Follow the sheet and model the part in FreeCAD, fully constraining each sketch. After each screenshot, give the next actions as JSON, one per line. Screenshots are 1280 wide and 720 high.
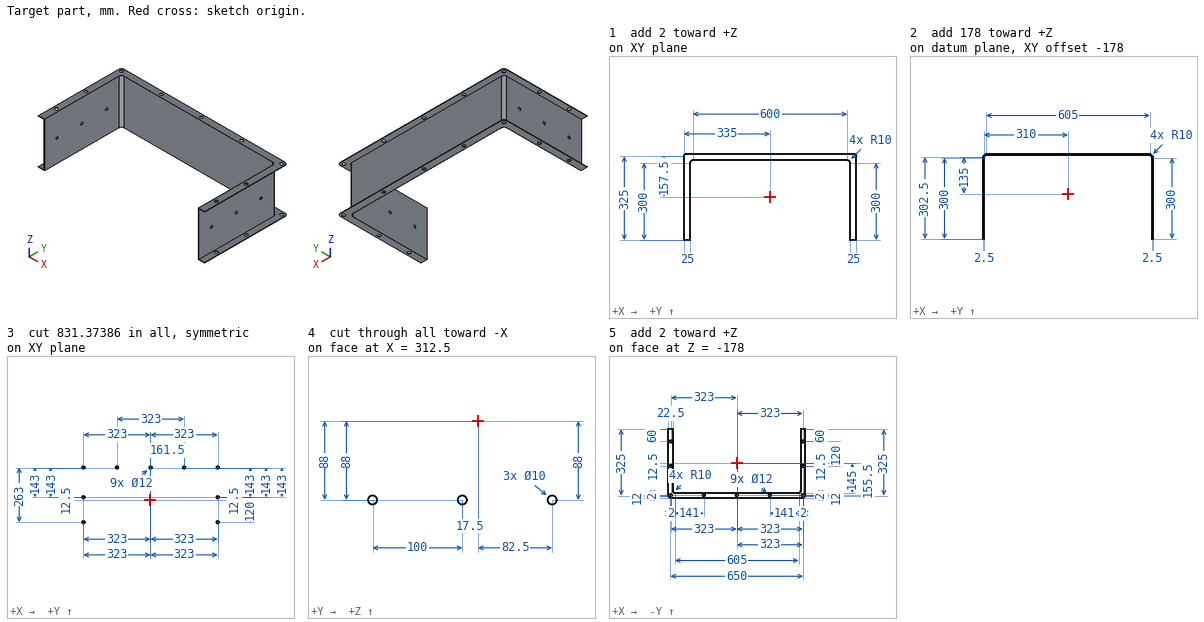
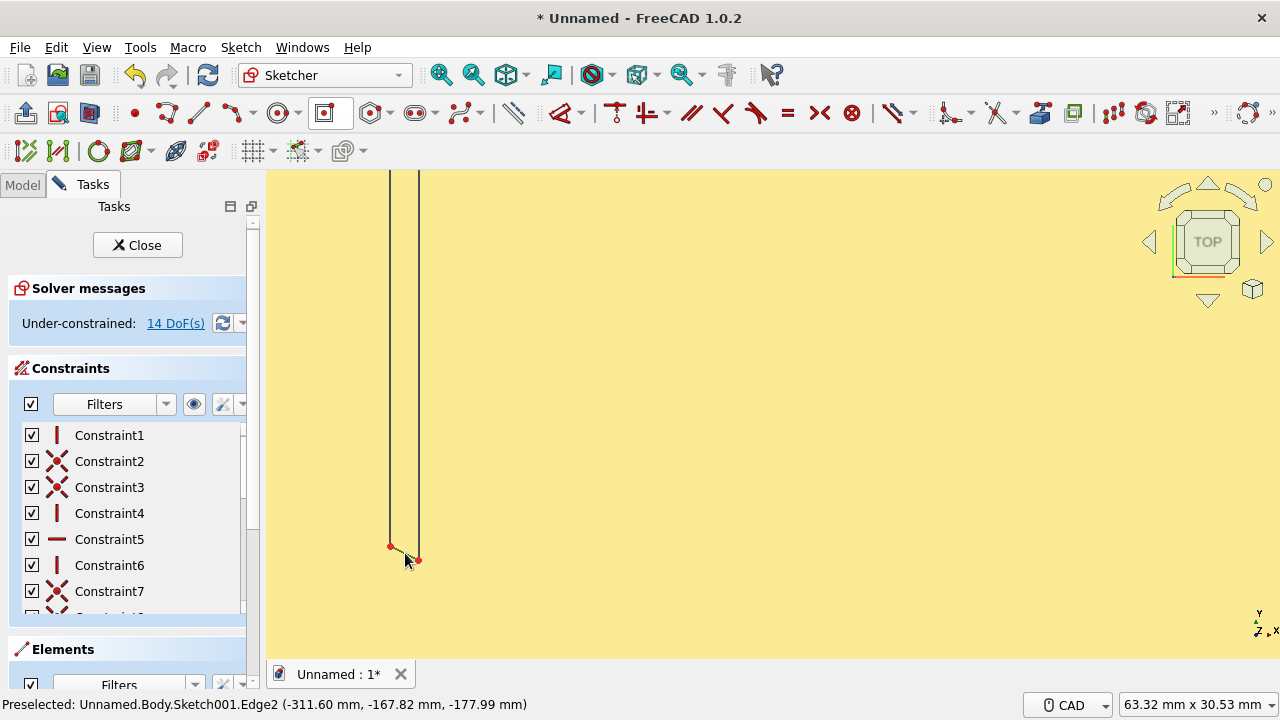
{"action": "left_click", "coordinate": [670, 114]}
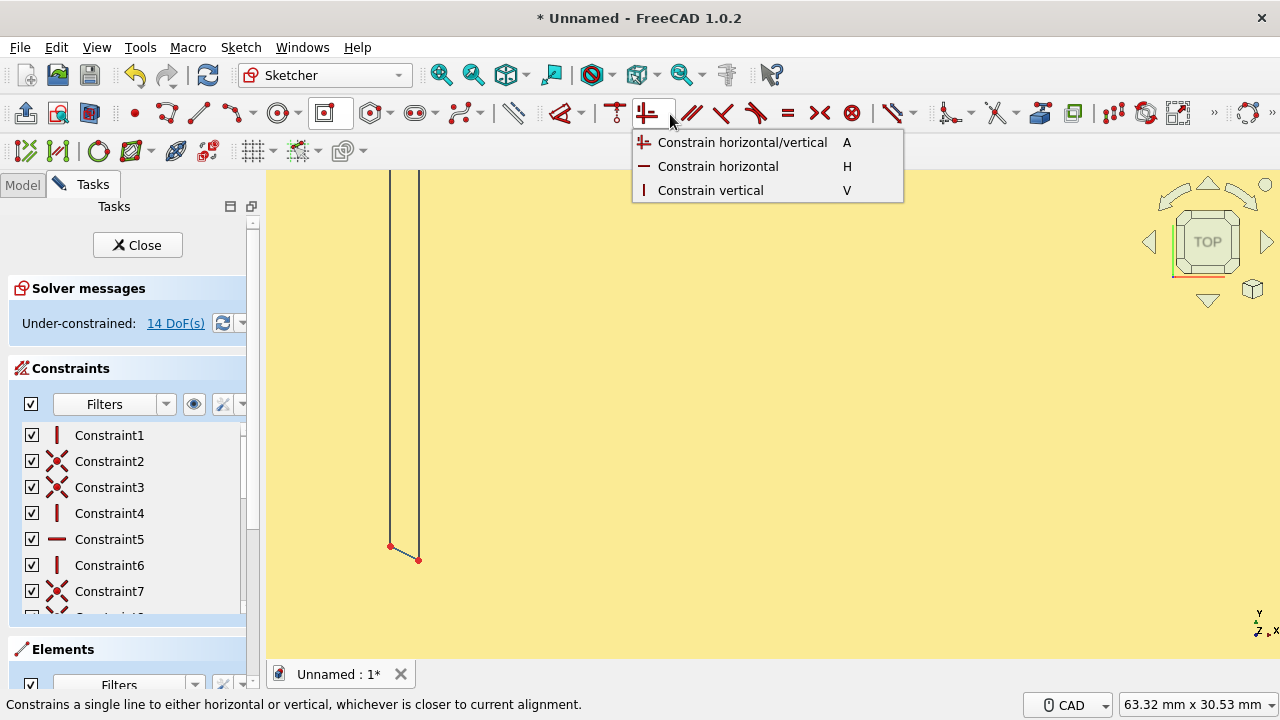
{"action": "left_click", "coordinate": [768, 166]}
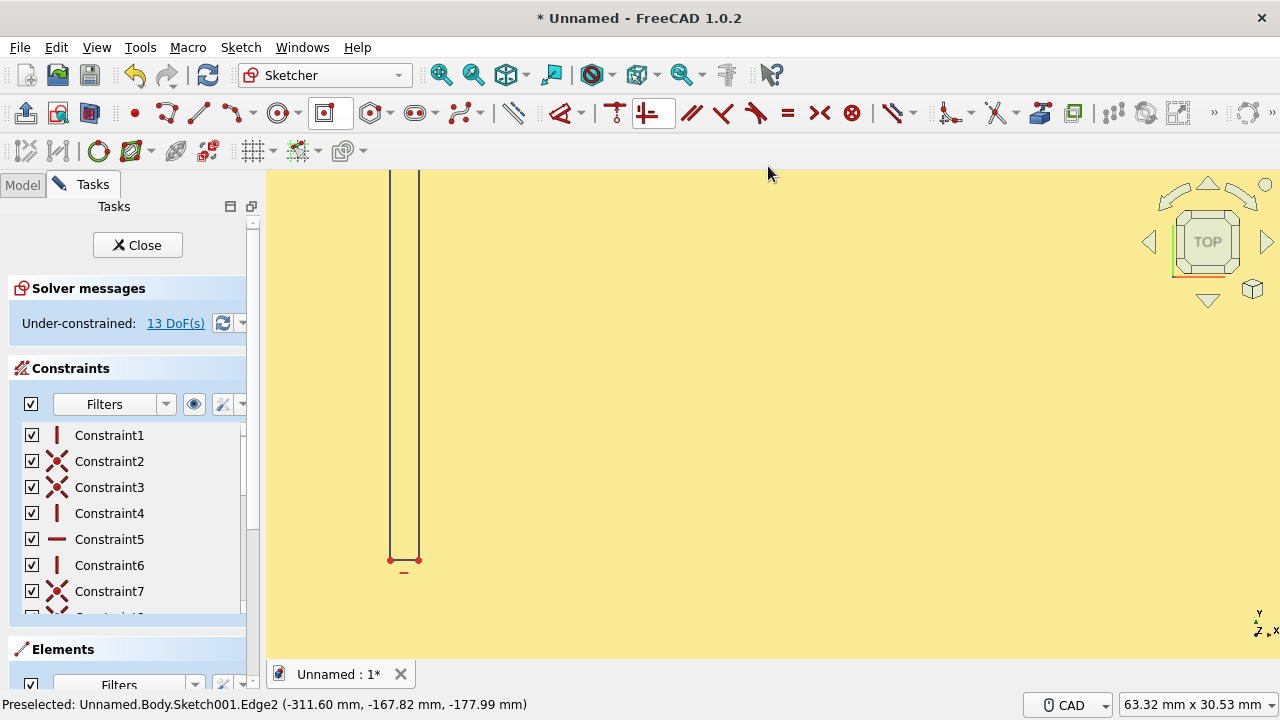
{"action": "scroll", "coordinate": [401, 568], "scroll_direction": "down", "scroll_amount": 14}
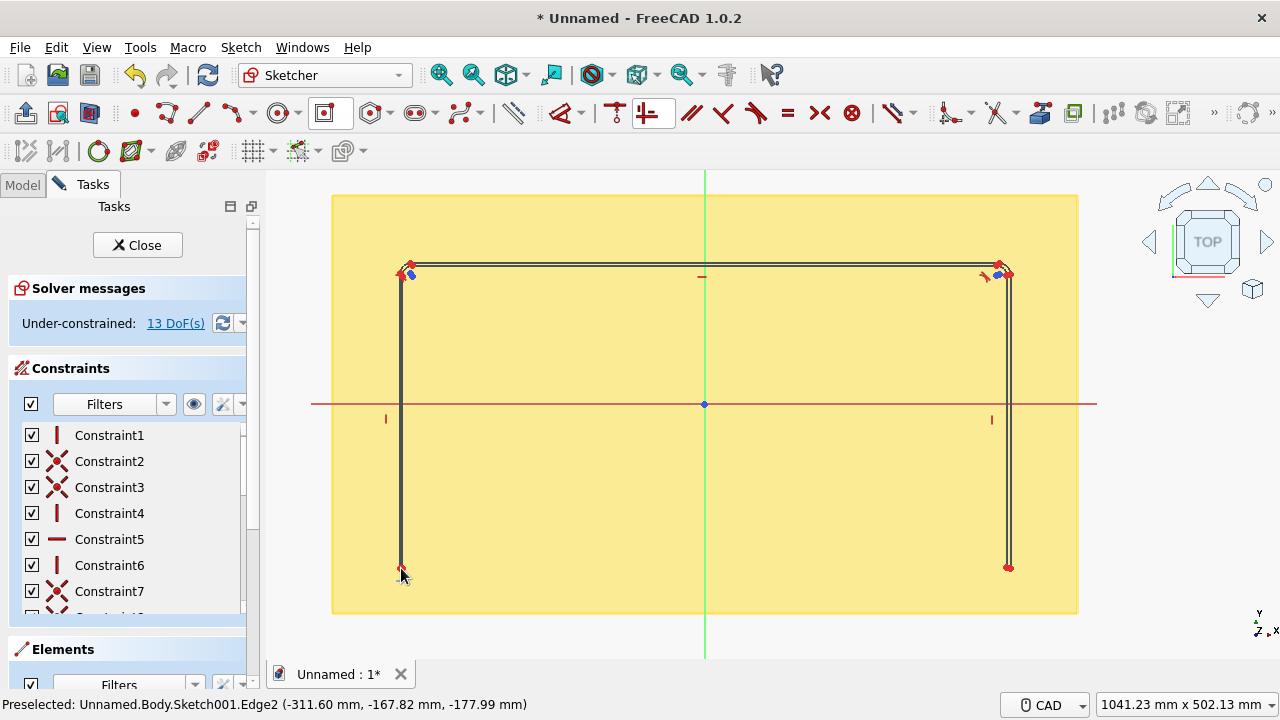
{"action": "scroll", "coordinate": [1009, 568], "scroll_direction": "up", "scroll_amount": 13}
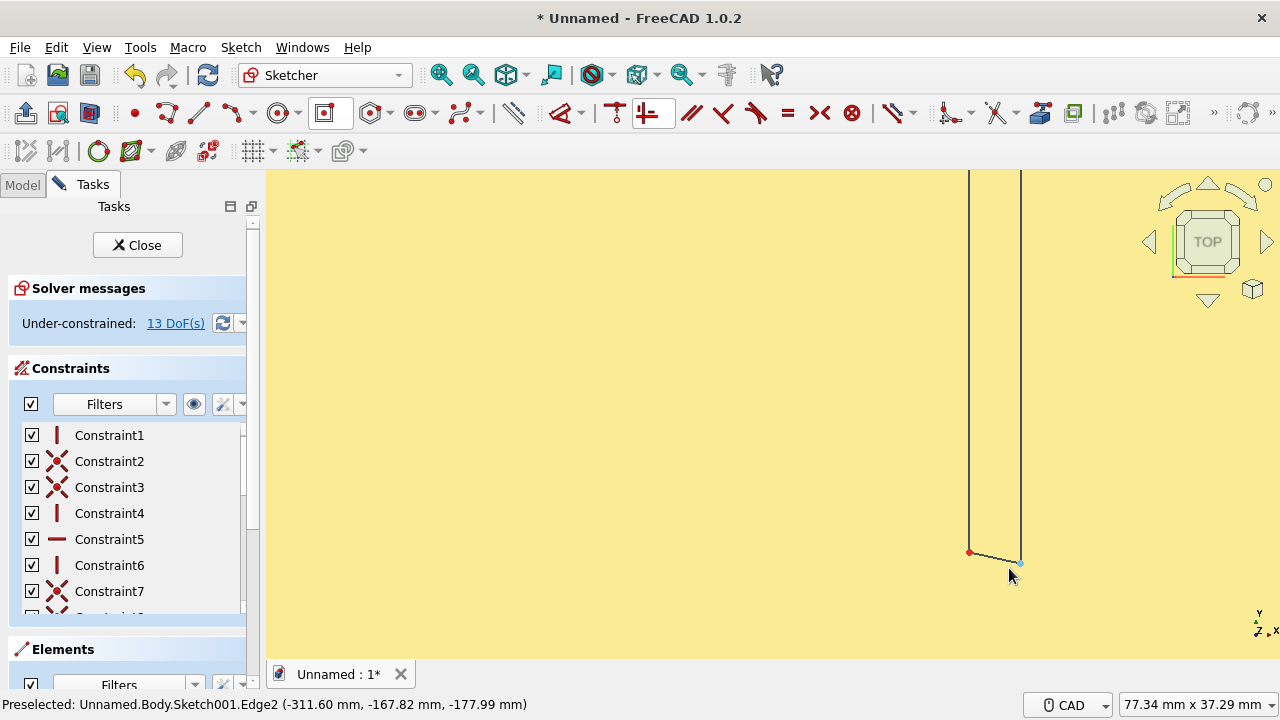
{"action": "left_click", "coordinate": [1005, 560]}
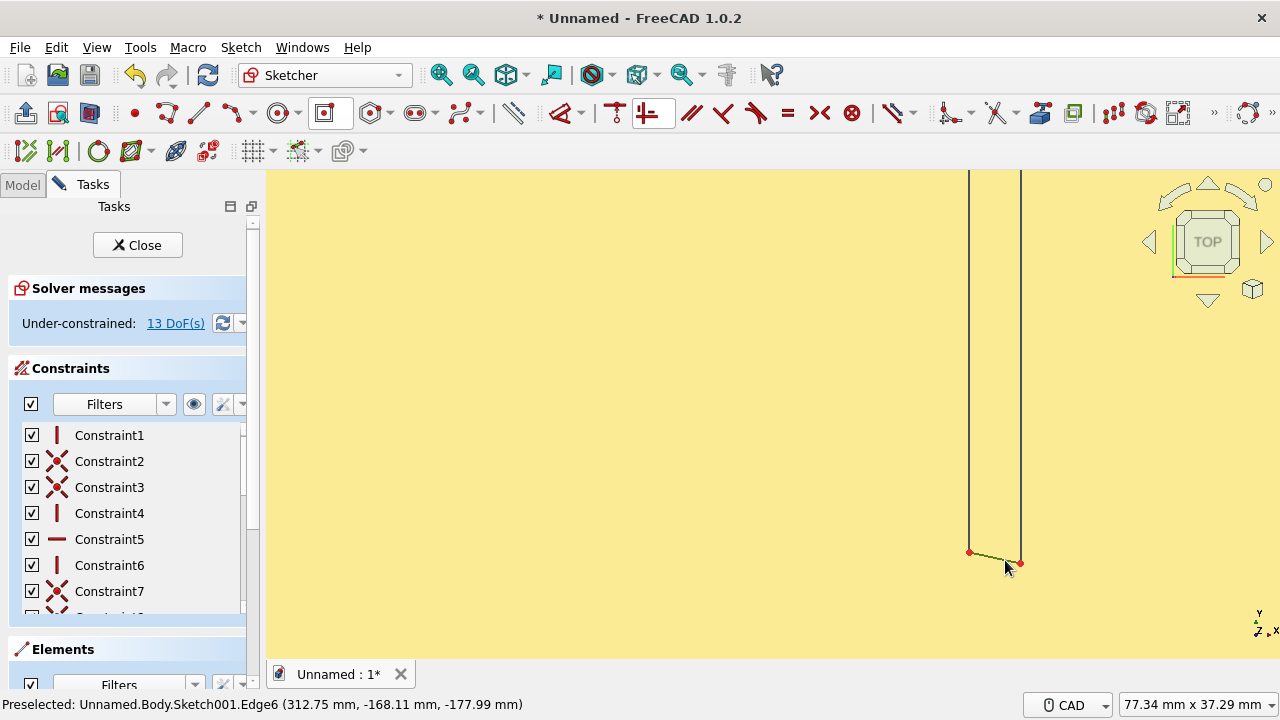
{"action": "left_click", "coordinate": [670, 114]}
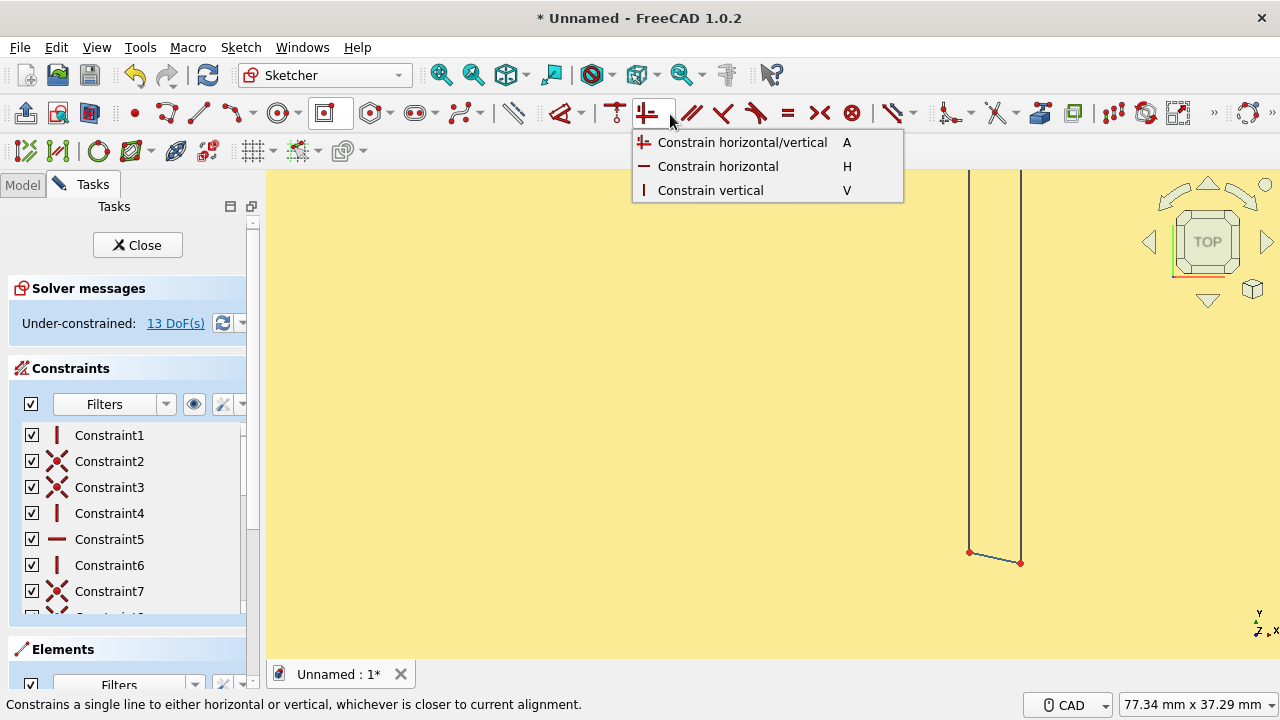
{"action": "left_click", "coordinate": [768, 166]}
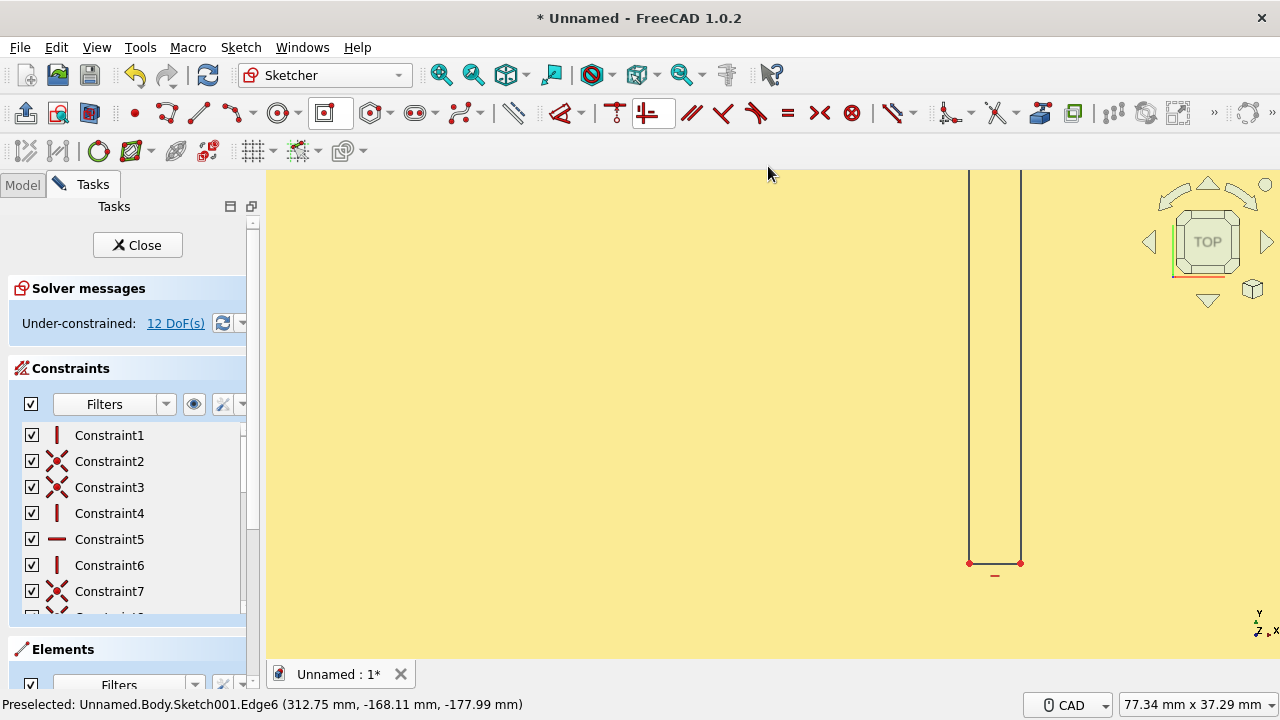
{"action": "scroll", "coordinate": [1009, 568], "scroll_direction": "down", "scroll_amount": 13}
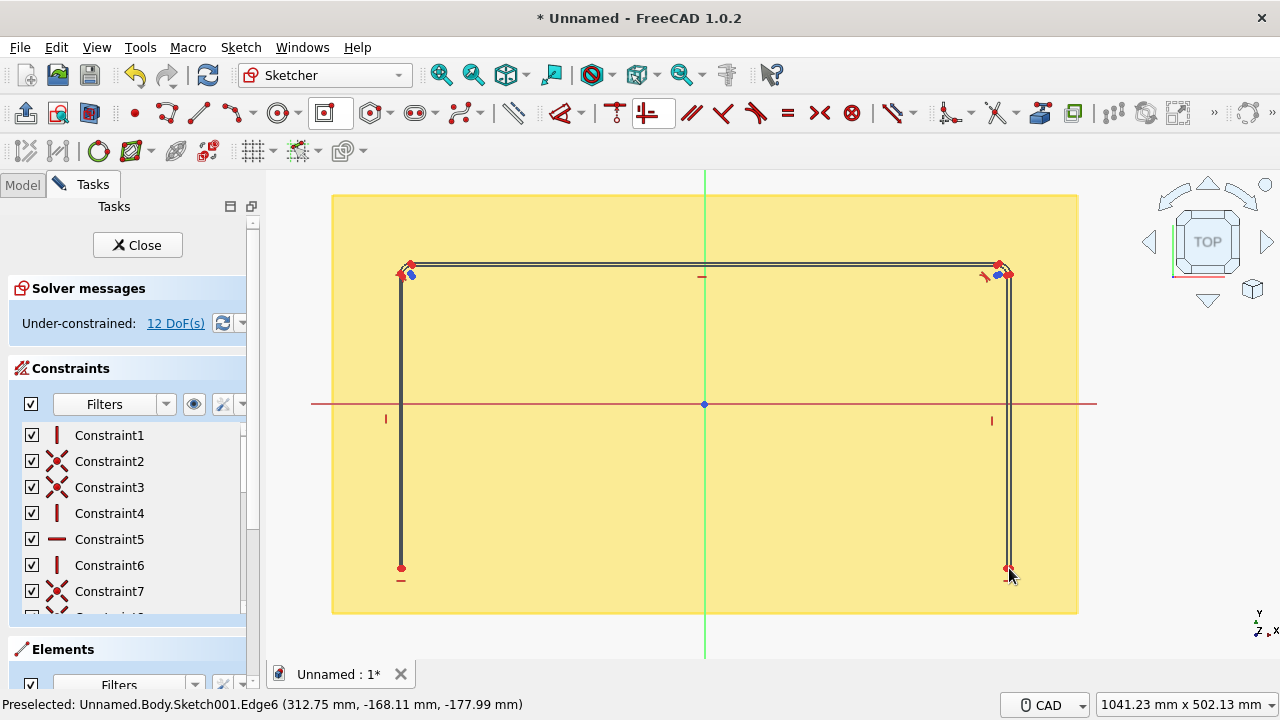
{"action": "scroll", "coordinate": [406, 264], "scroll_direction": "up", "scroll_amount": 8}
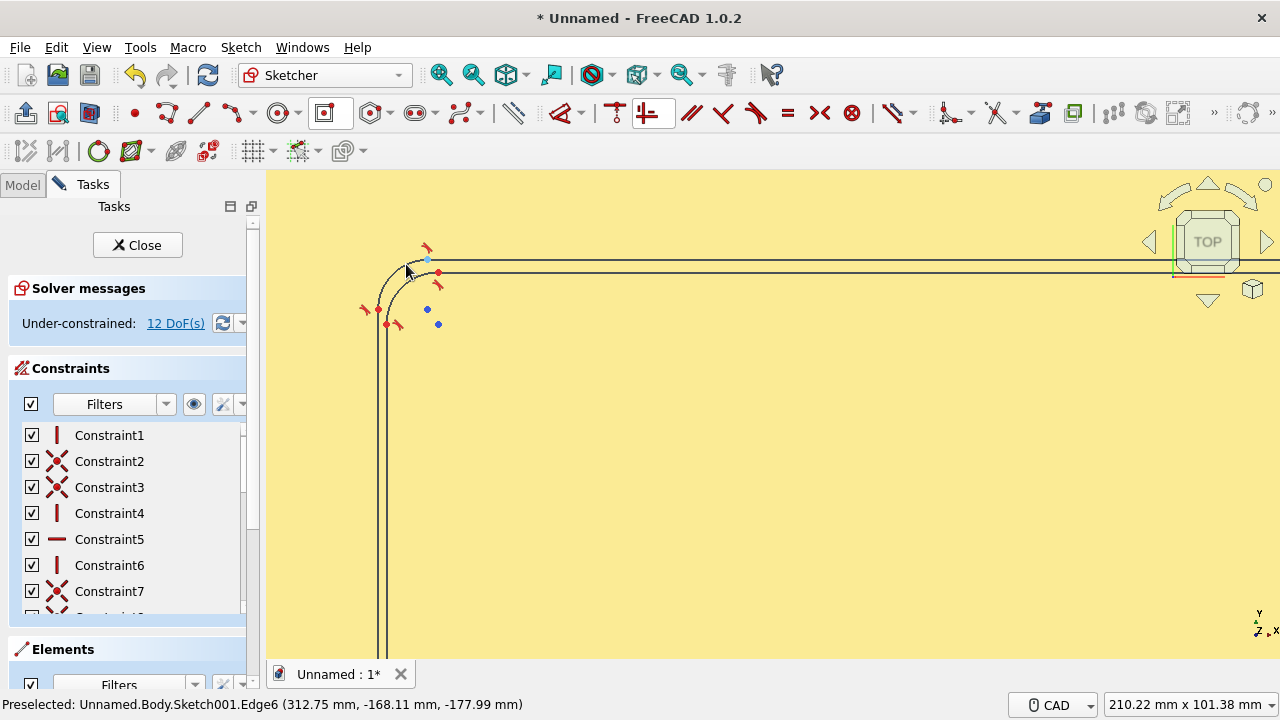
{"action": "left_click", "coordinate": [405, 265]}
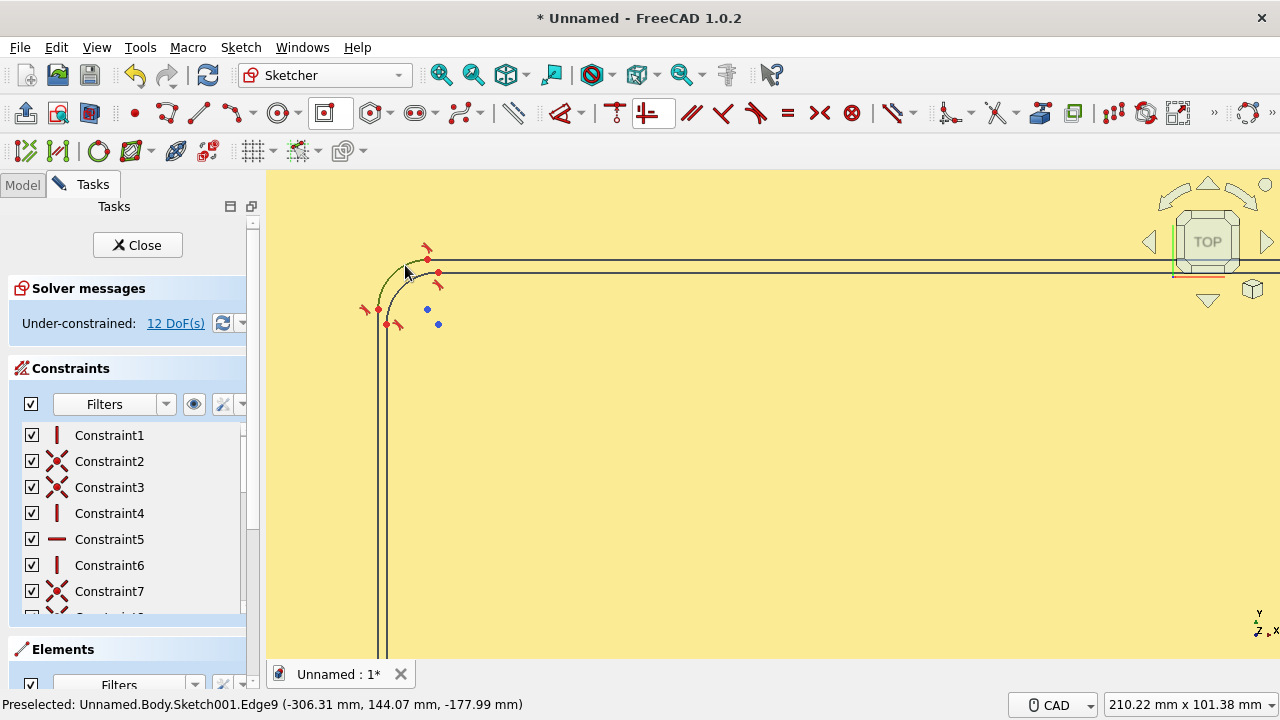
{"action": "scroll", "coordinate": [406, 263], "scroll_direction": "down", "scroll_amount": 8}